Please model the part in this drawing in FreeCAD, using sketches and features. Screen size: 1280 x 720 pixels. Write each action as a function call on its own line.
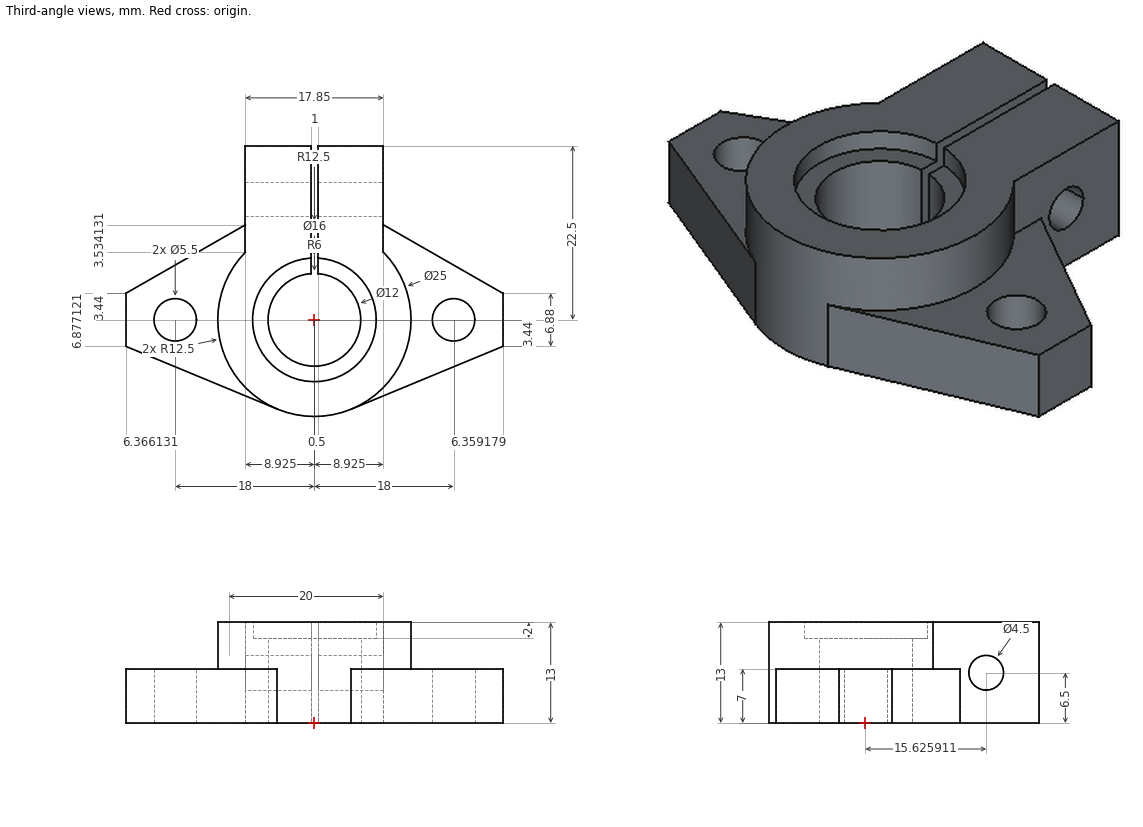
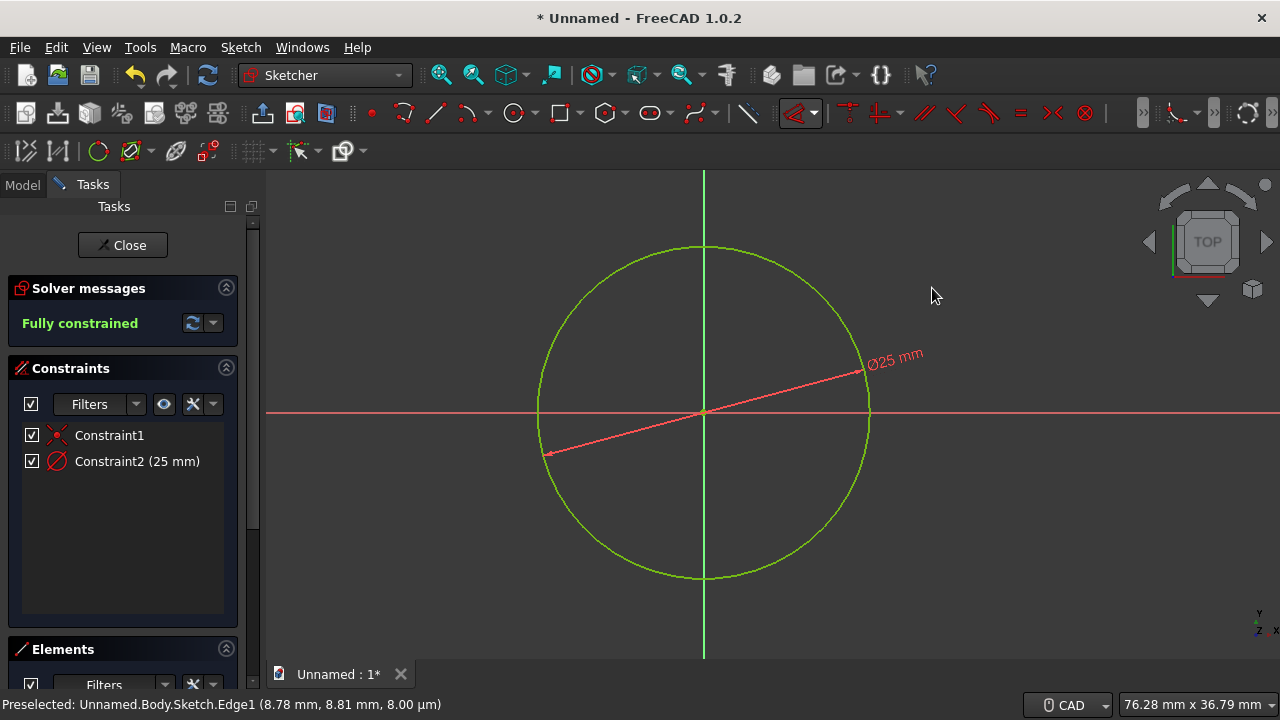
click(123, 245)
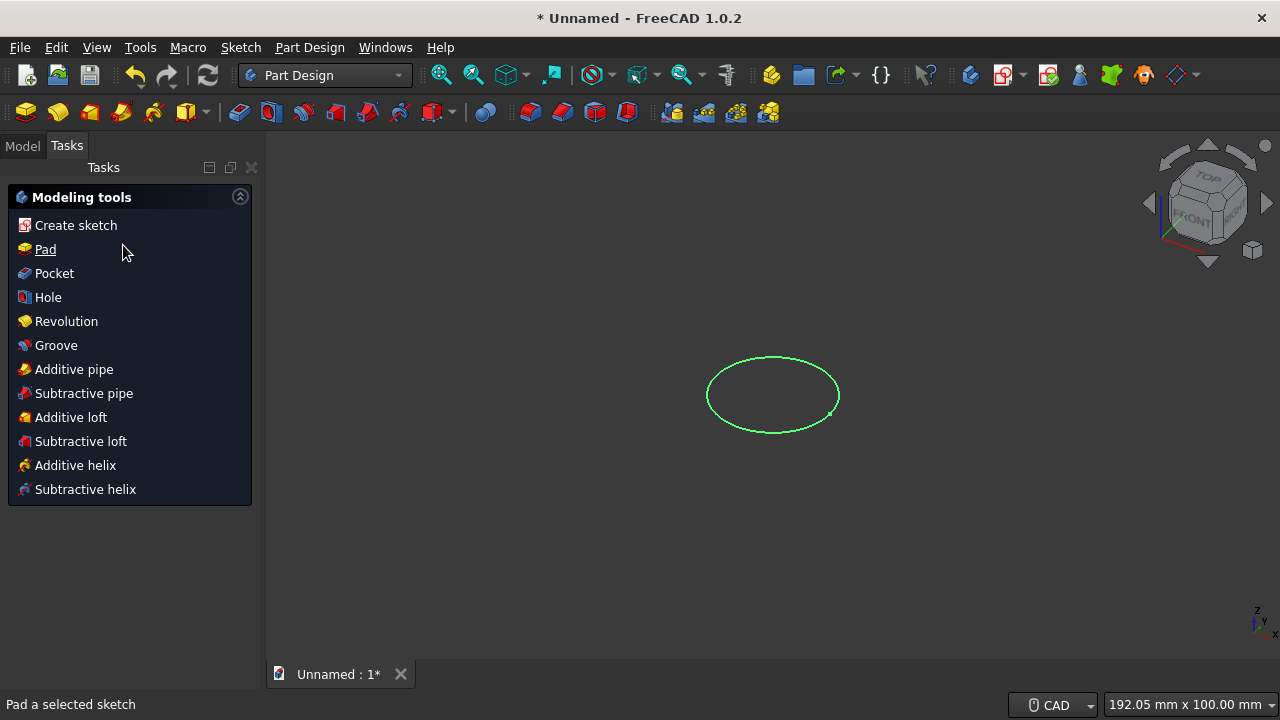
click(26, 112)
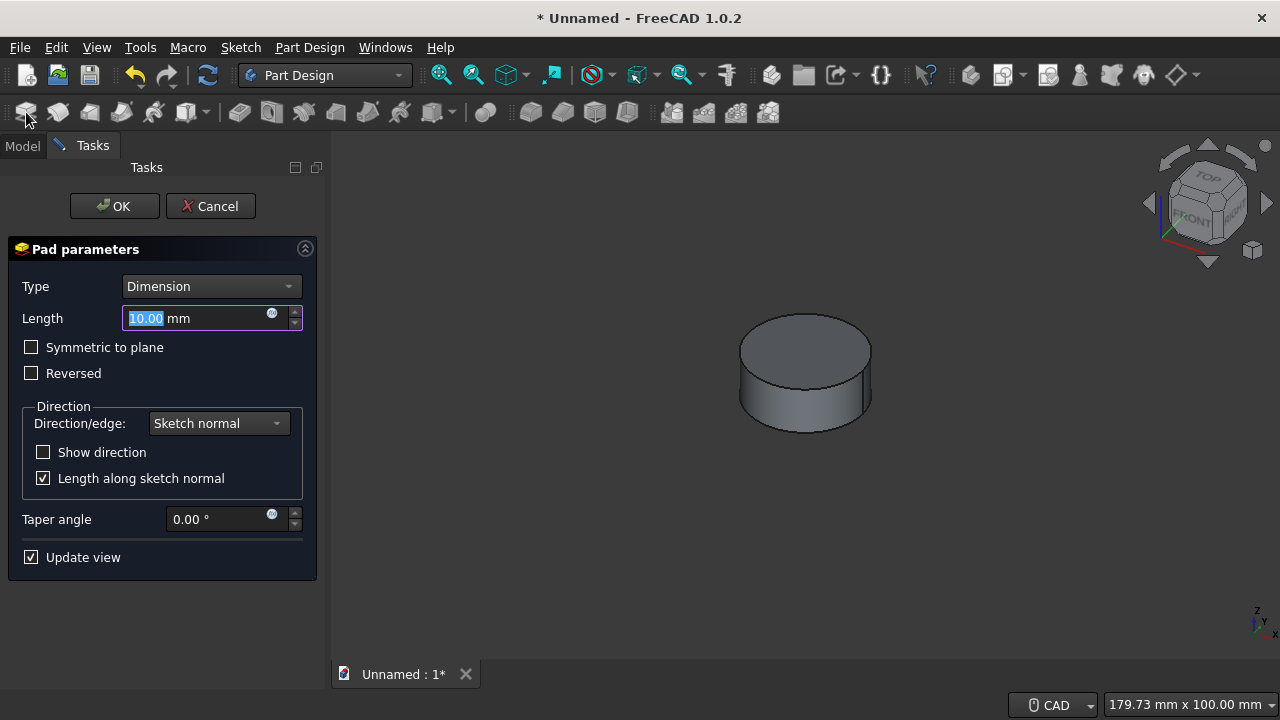
text(13)
key(Tab)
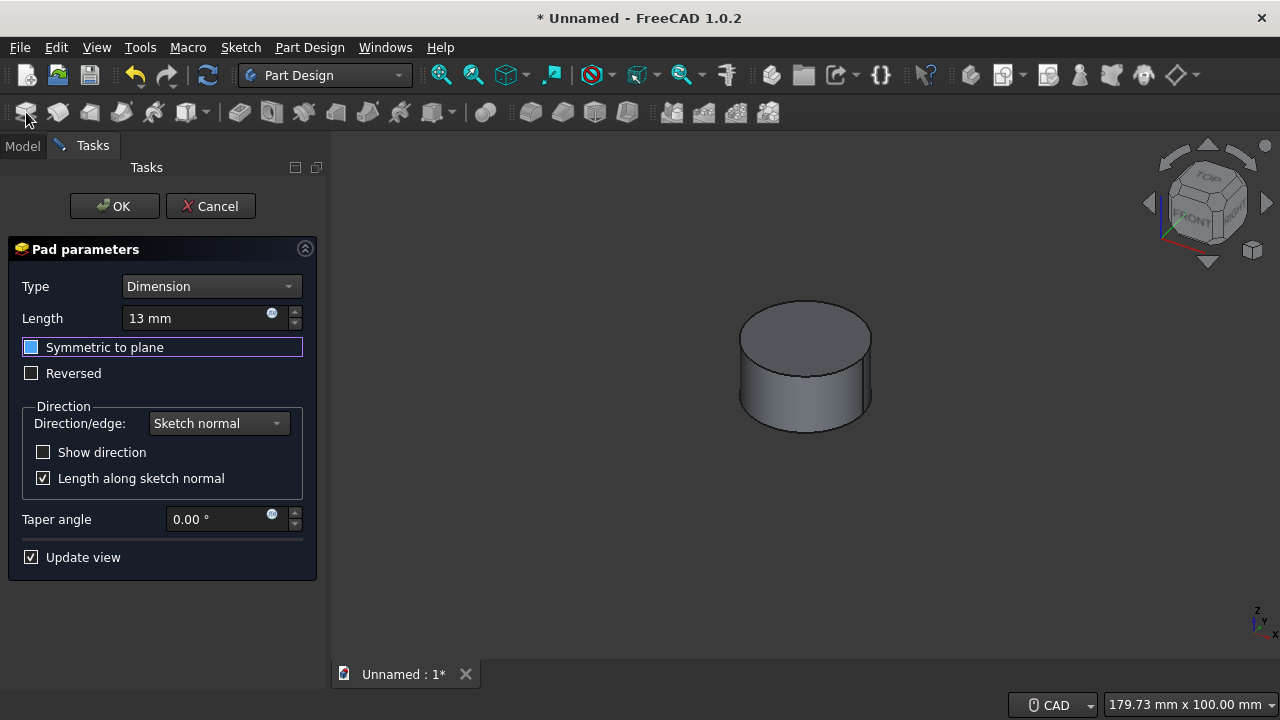
click(115, 206)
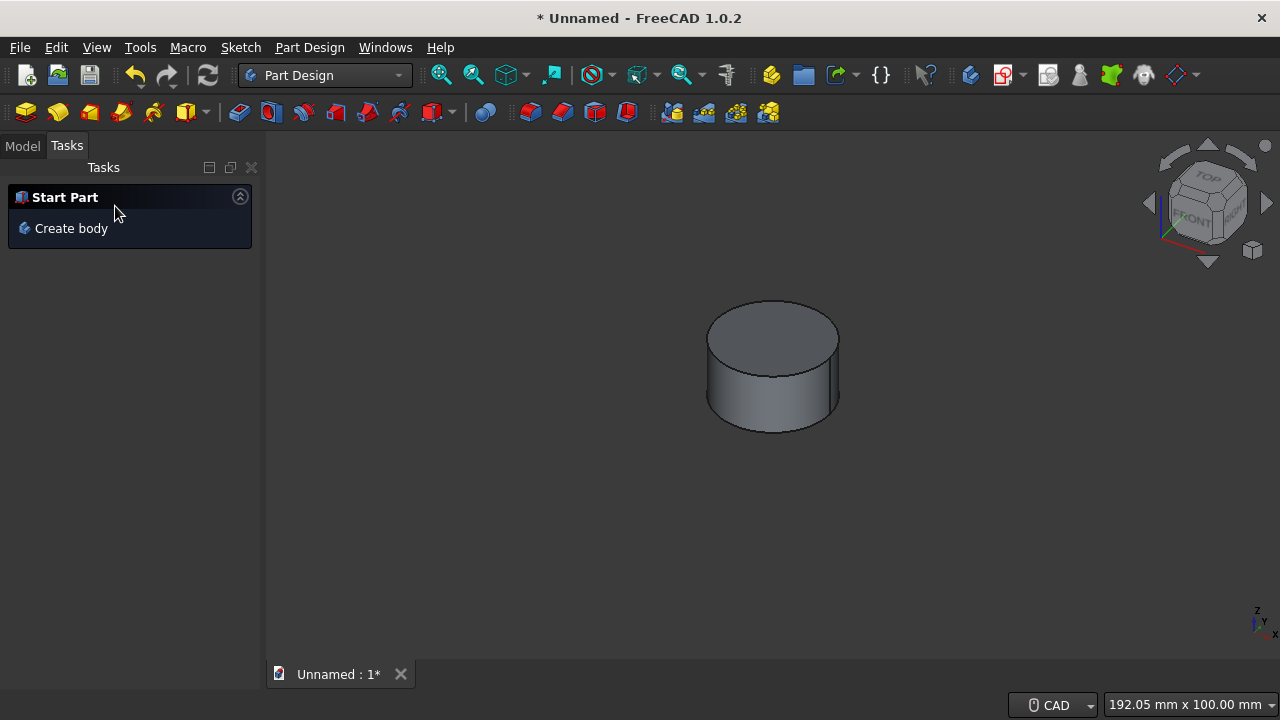
click(442, 76)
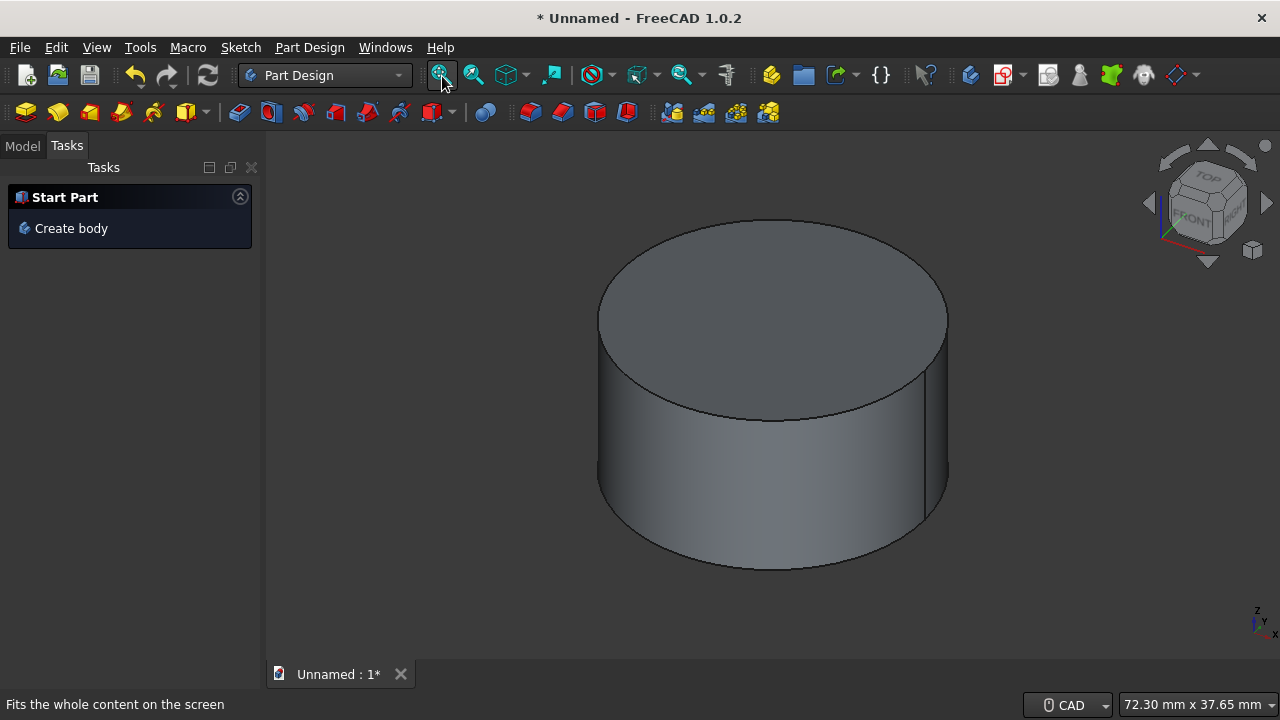
click(1004, 76)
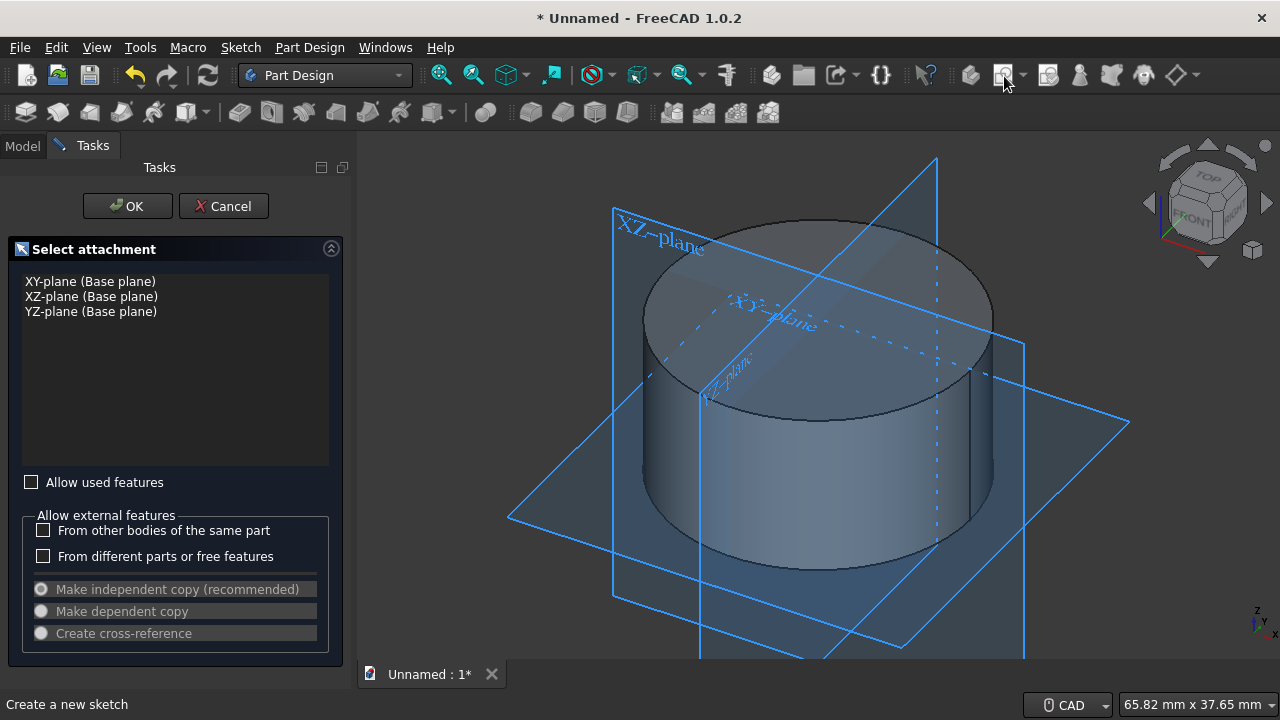
click(82, 282)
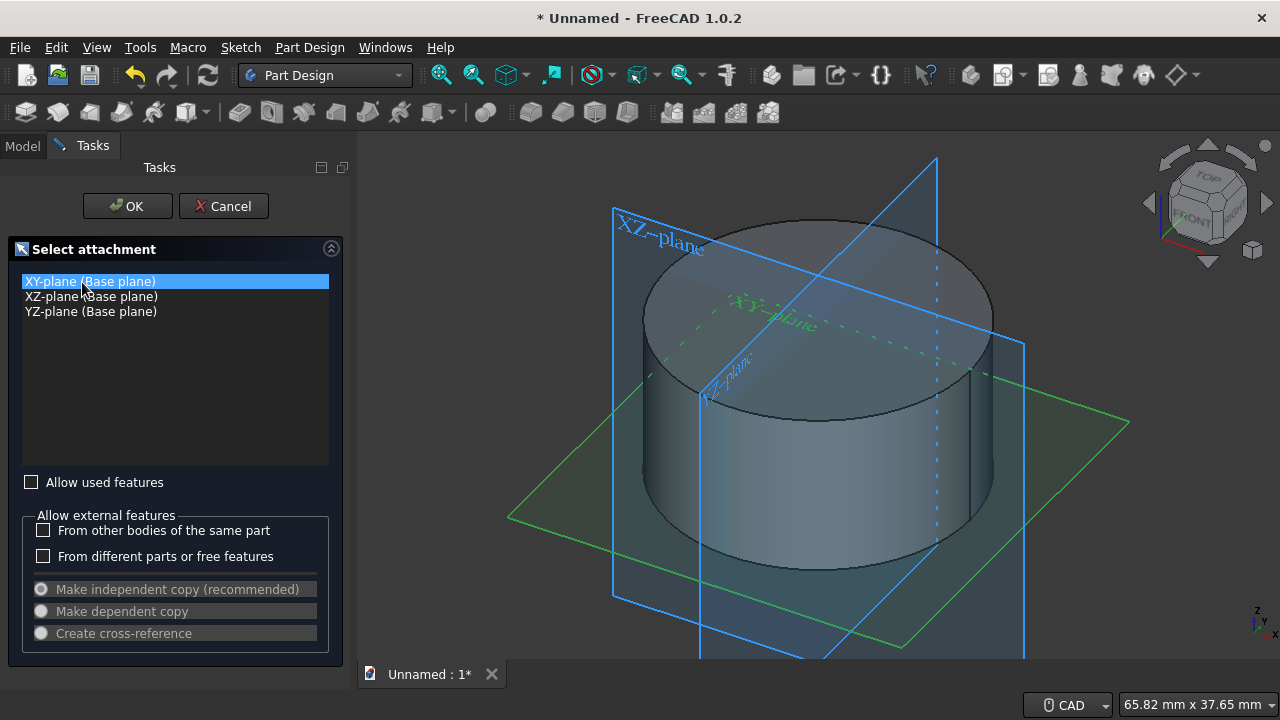
click(128, 206)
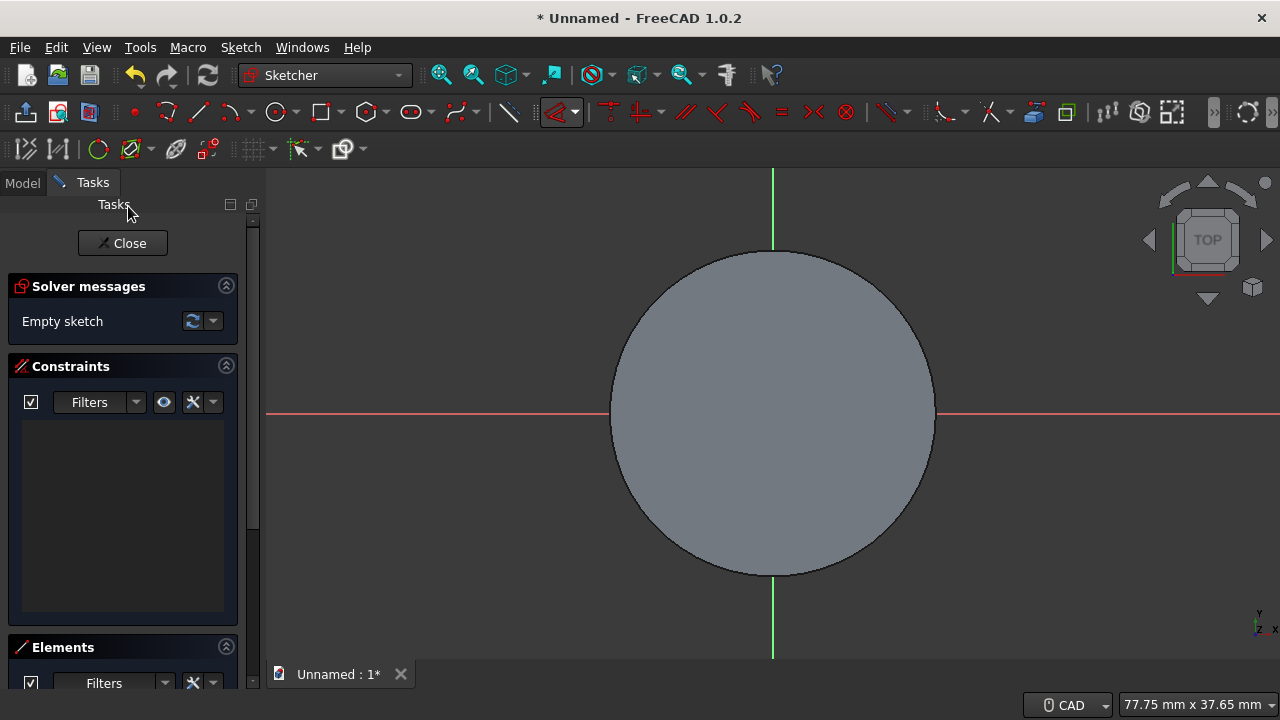
click(90, 112)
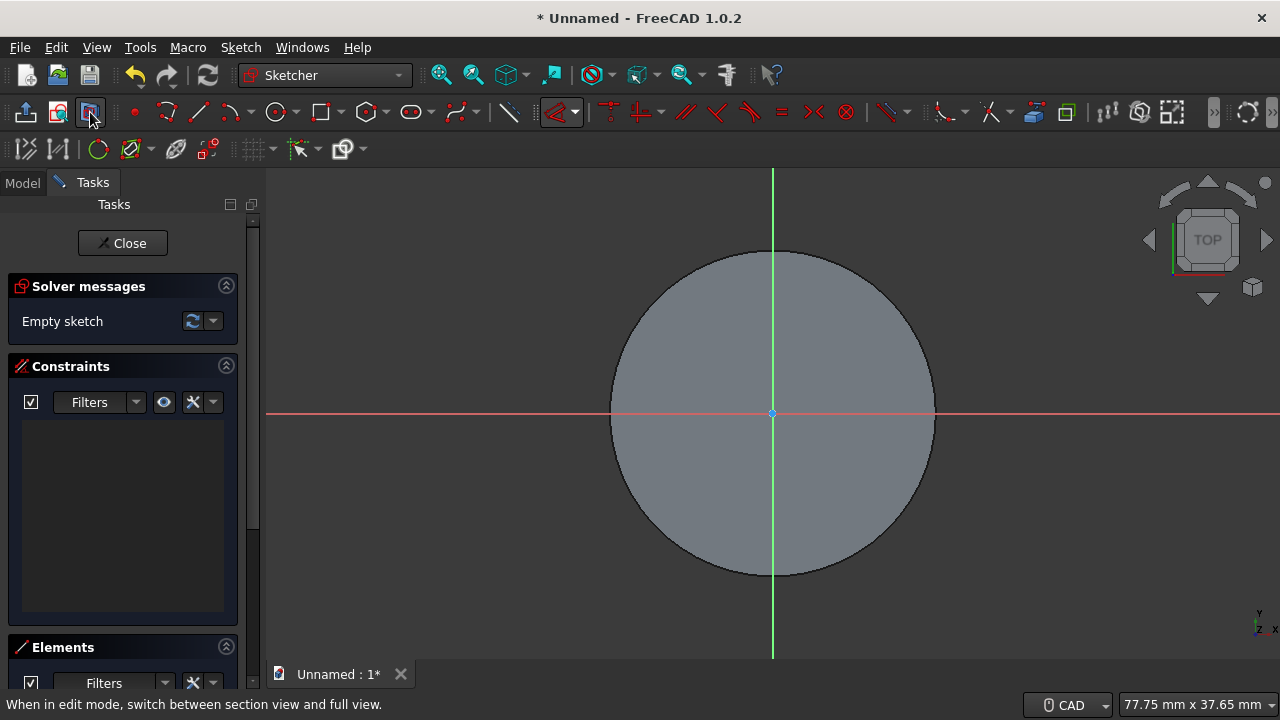
scroll(565, 631, down, 2)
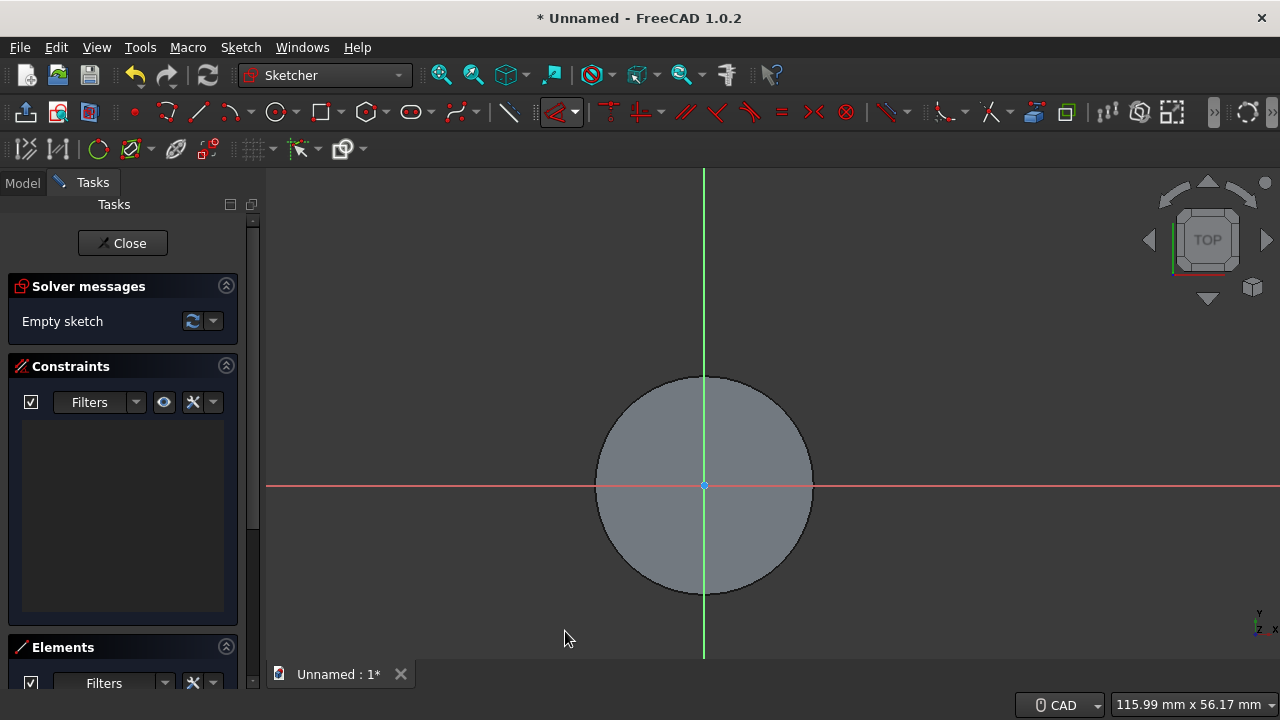
scroll(704, 334, up, 2)